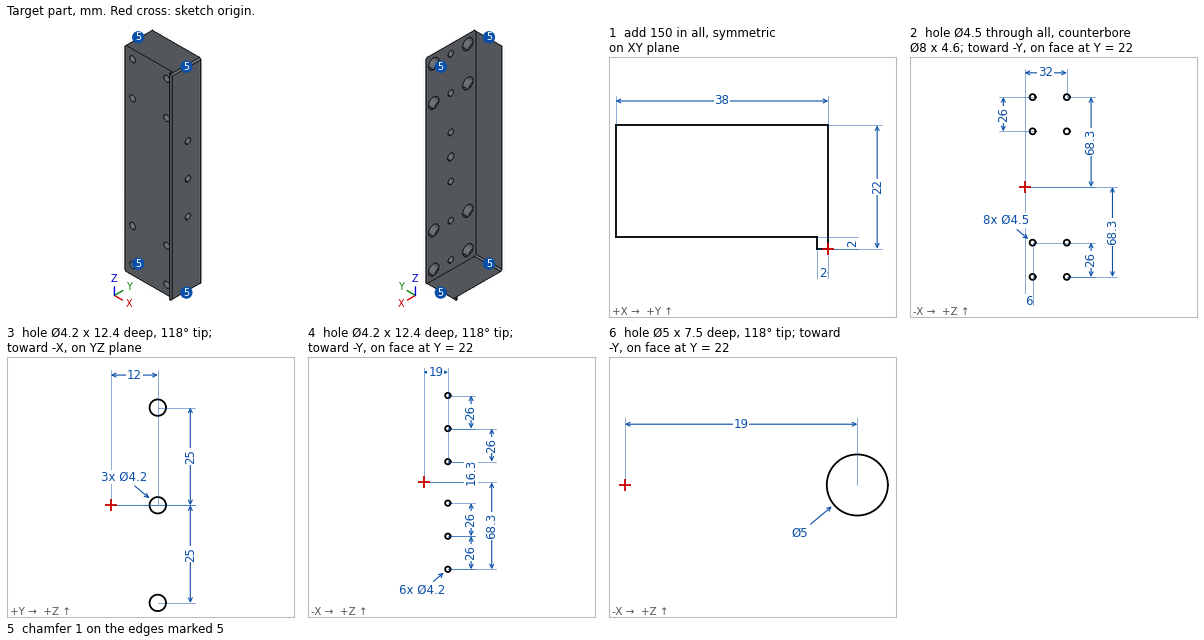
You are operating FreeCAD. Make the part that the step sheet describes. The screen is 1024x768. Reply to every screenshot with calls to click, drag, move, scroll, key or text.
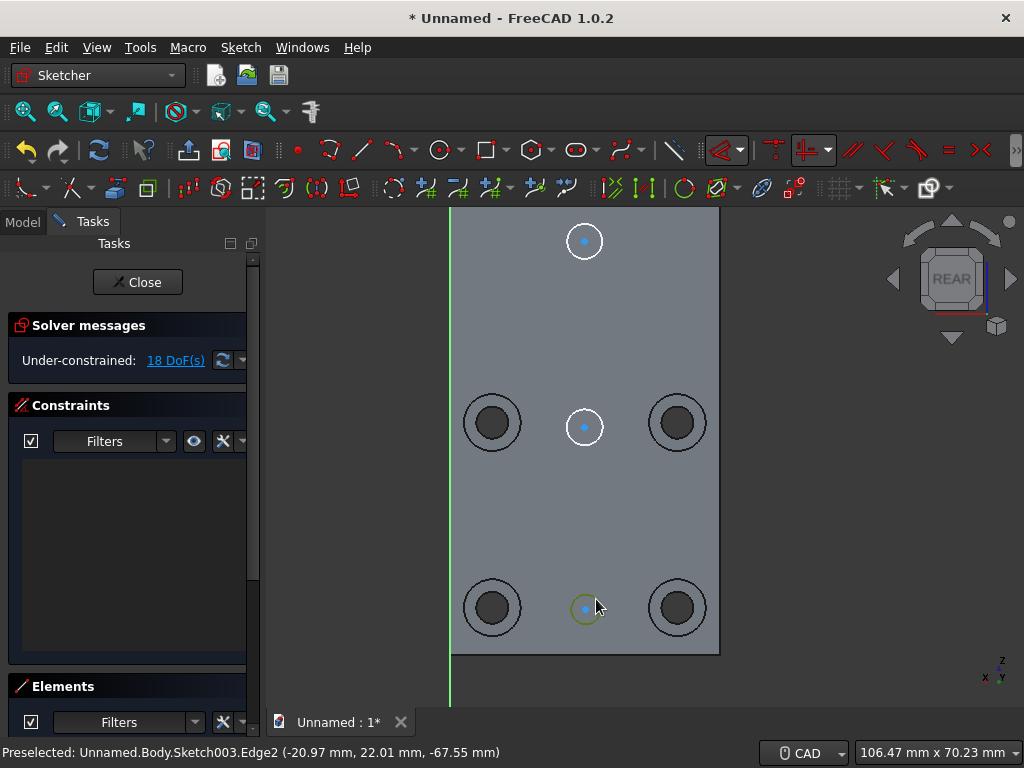
click(597, 415)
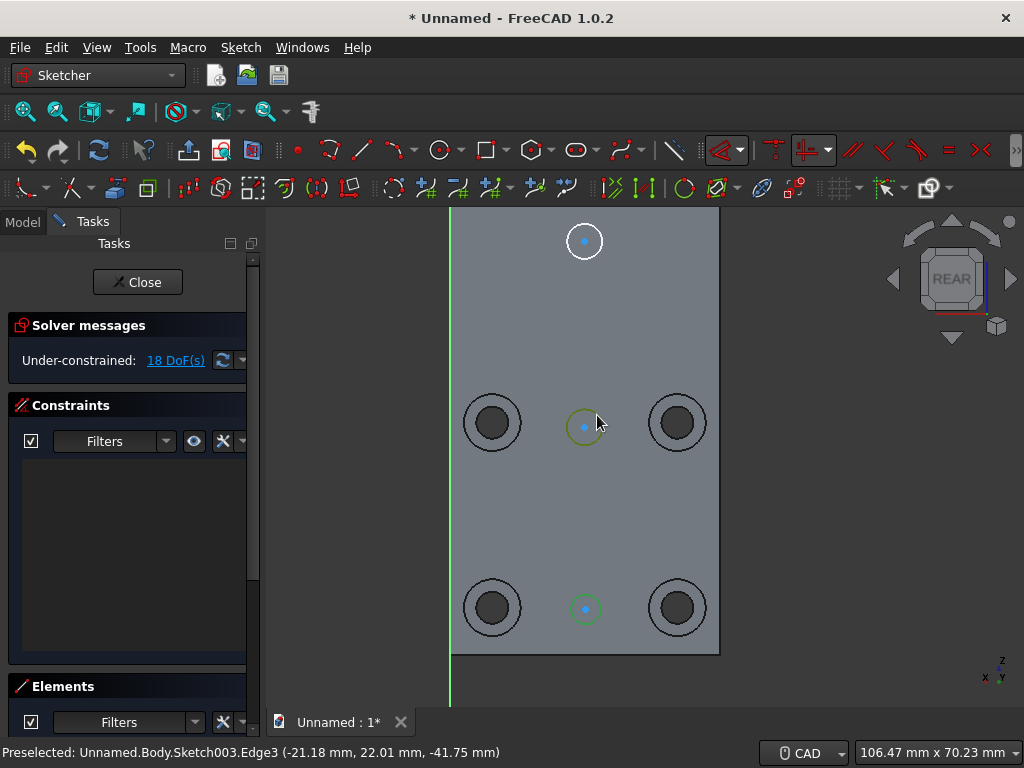
scroll(599, 602, down, 6)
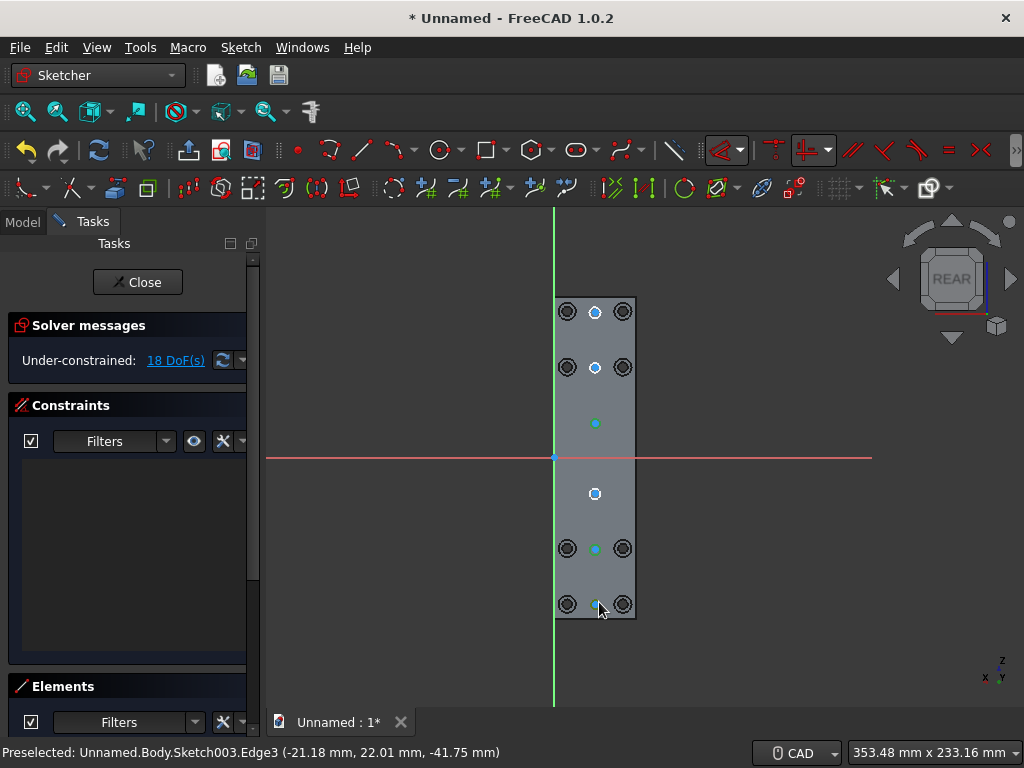
scroll(598, 364, up, 6)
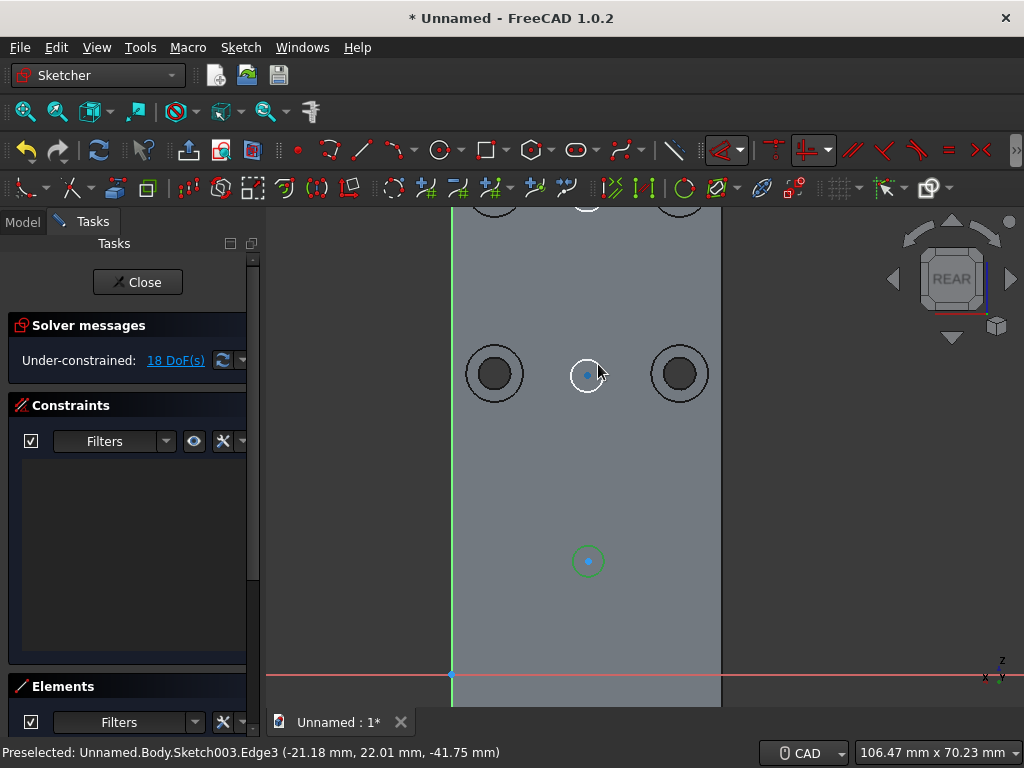
click(598, 364)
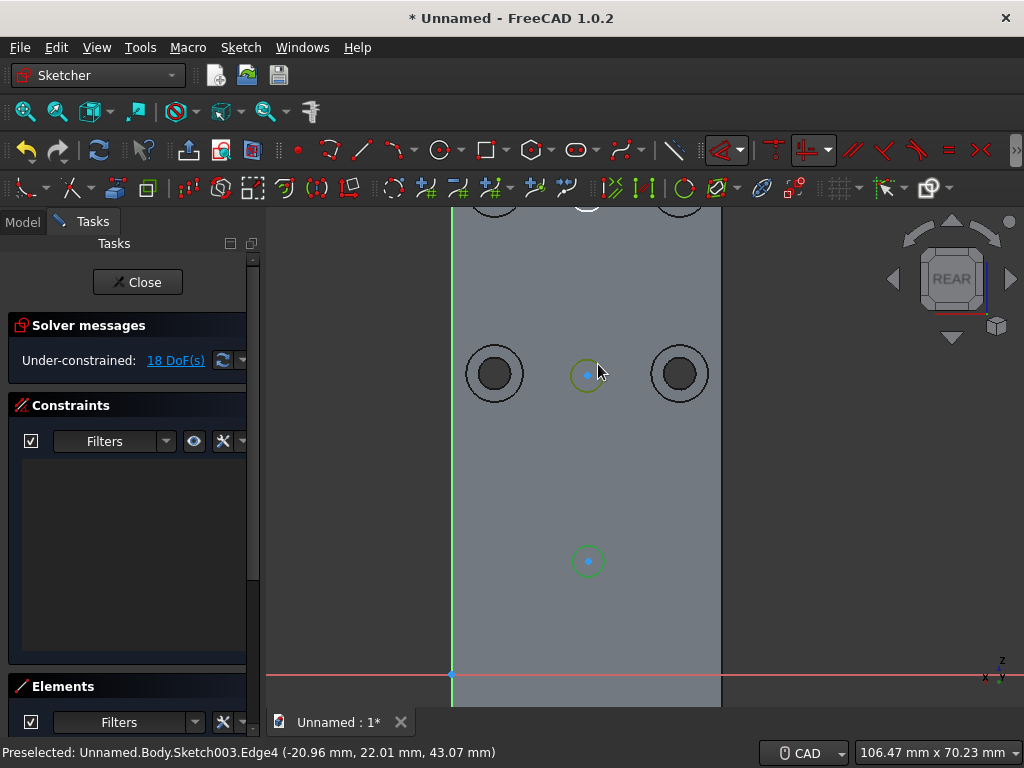
scroll(598, 363, down, 6)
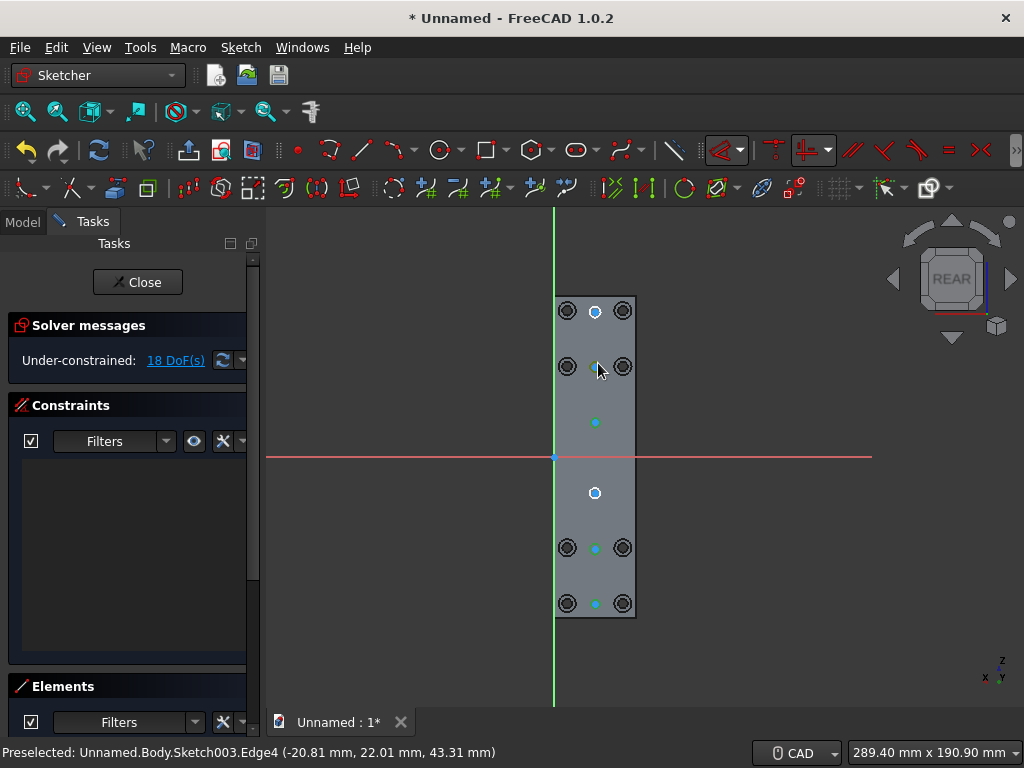
scroll(599, 308, up, 5)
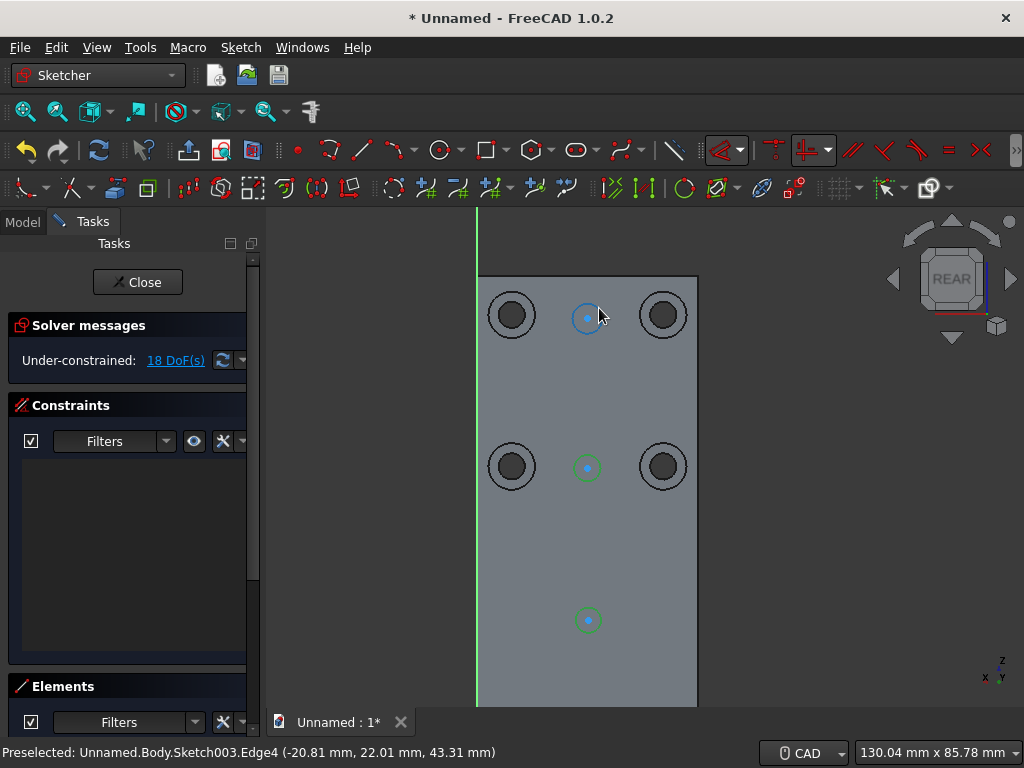
click(598, 308)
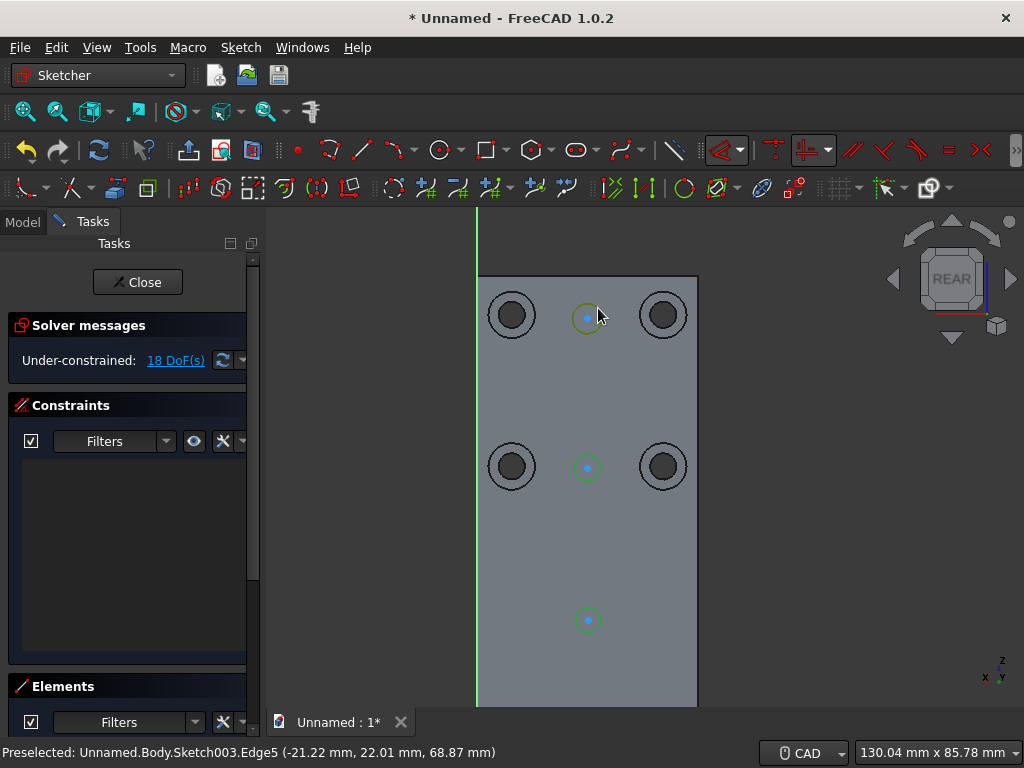
scroll(599, 308, down, 5)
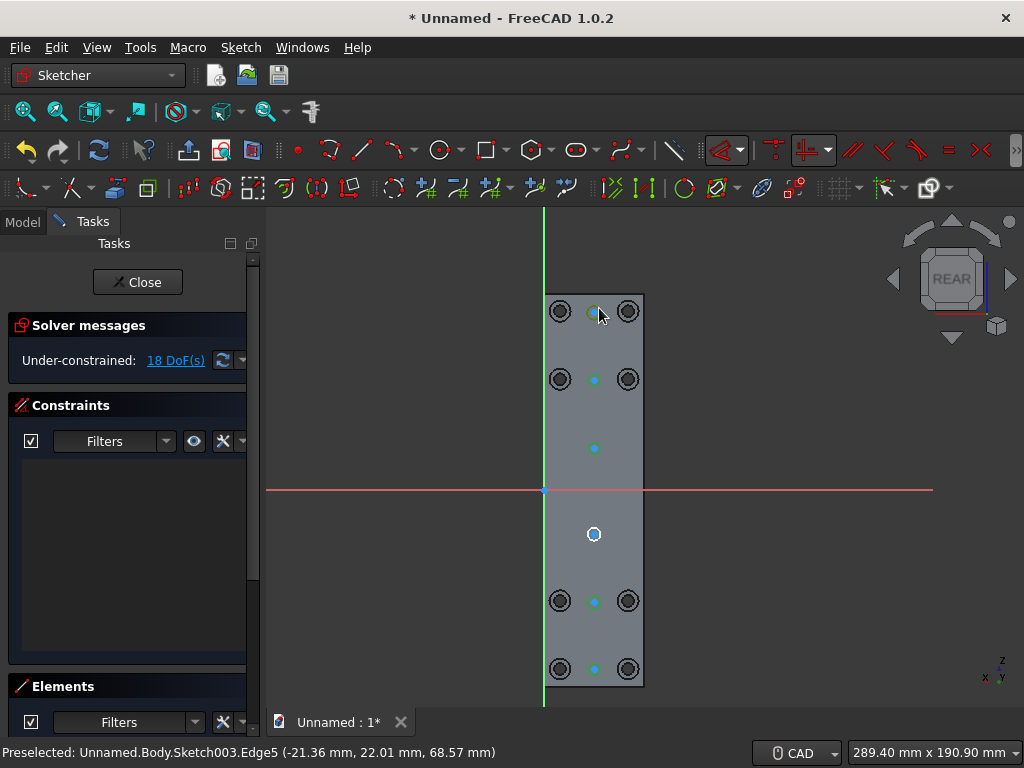
scroll(599, 490, up, 5)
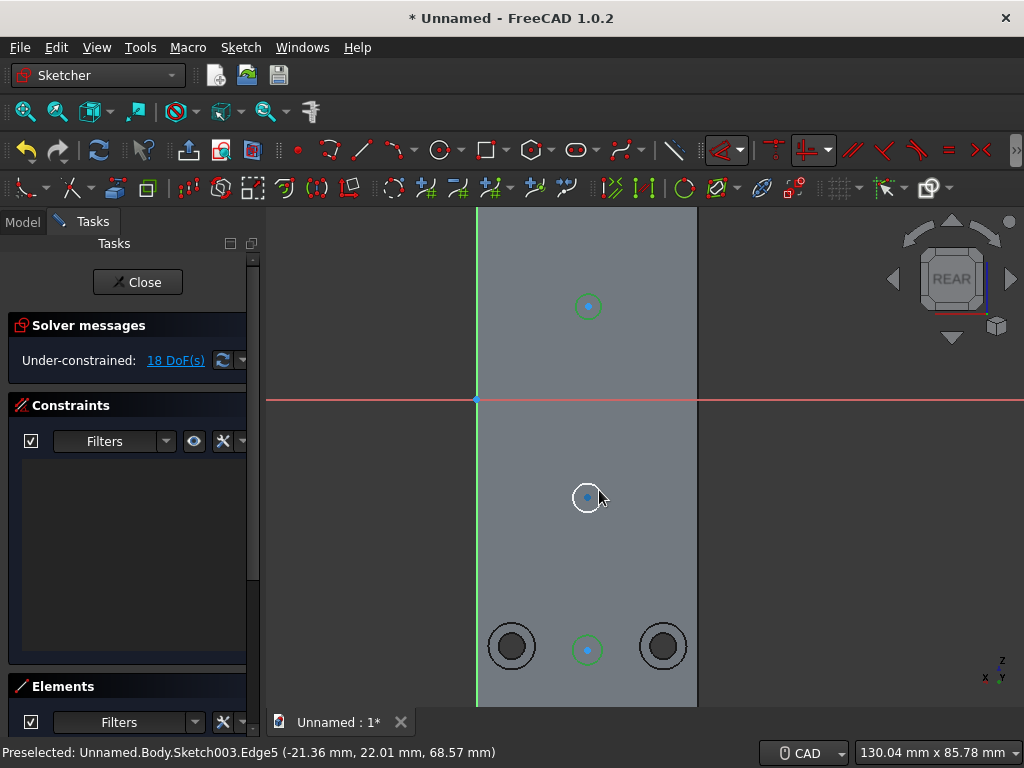
click(597, 488)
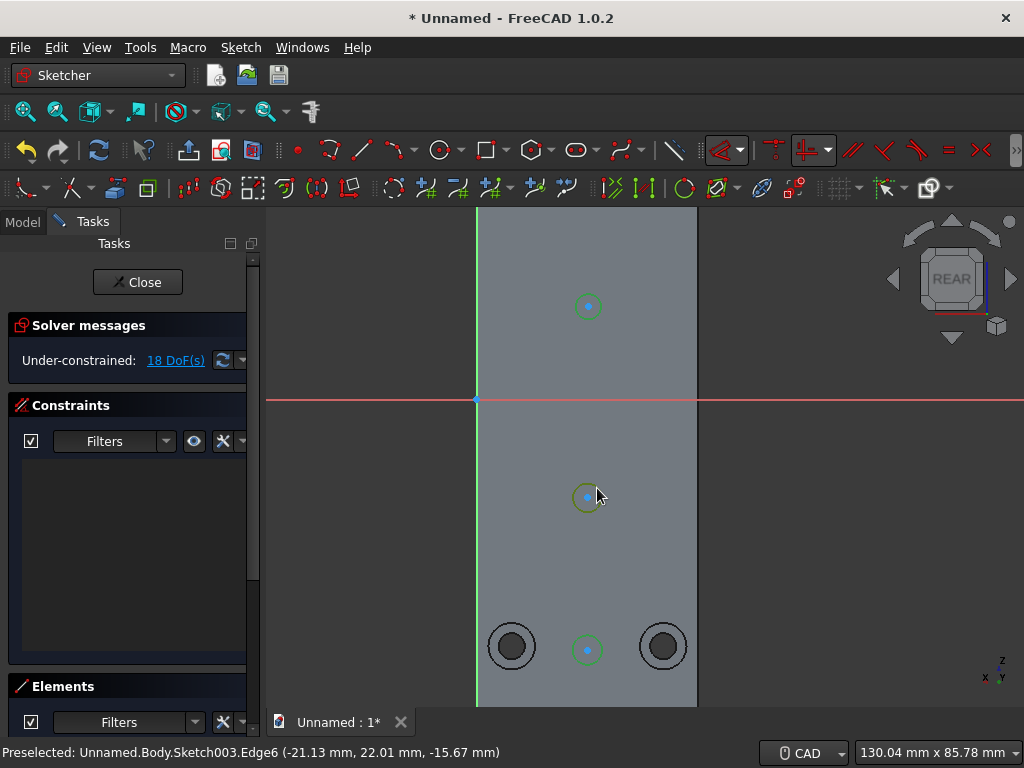
click(950, 150)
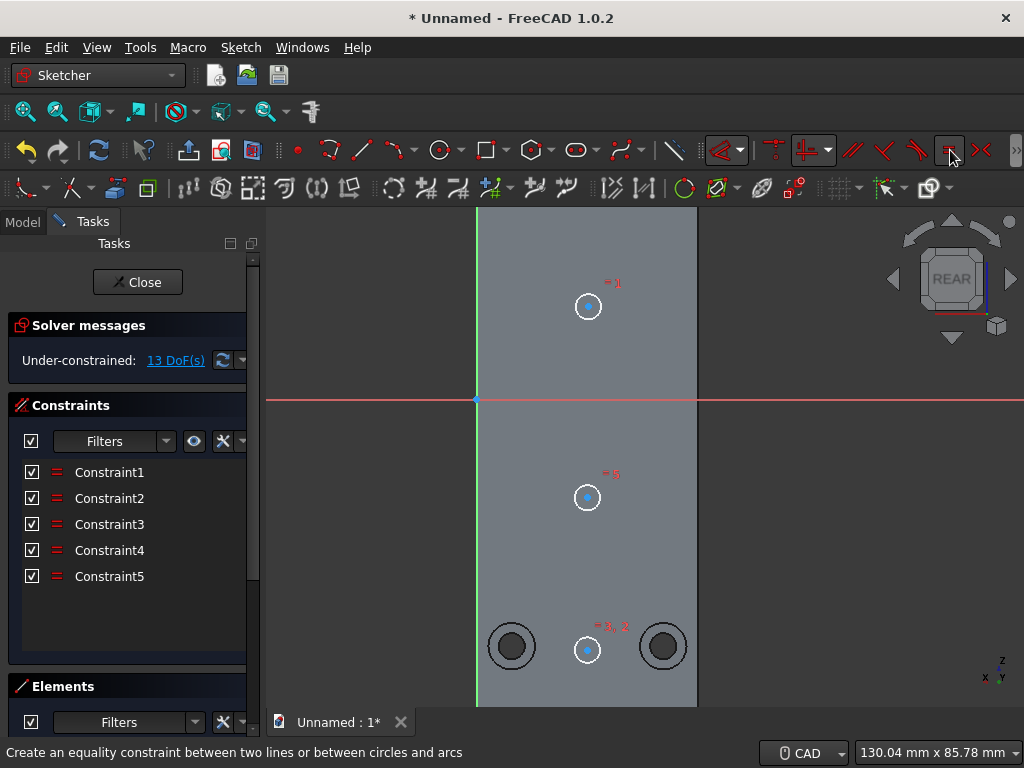
click(588, 307)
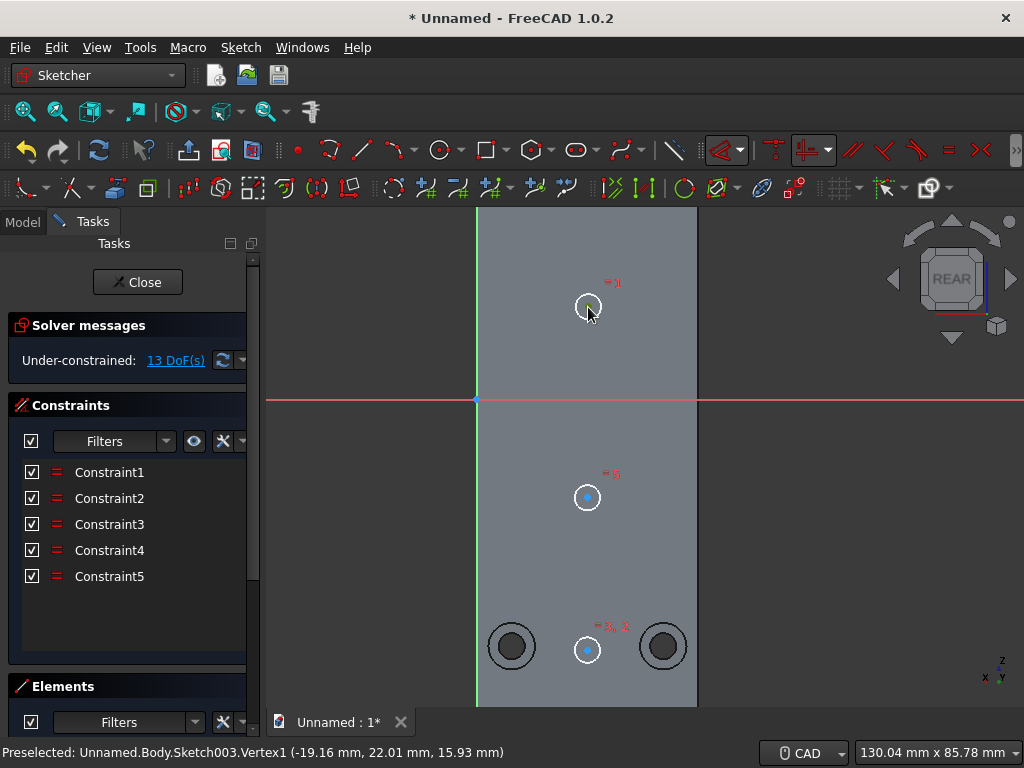
scroll(599, 490, down, 5)